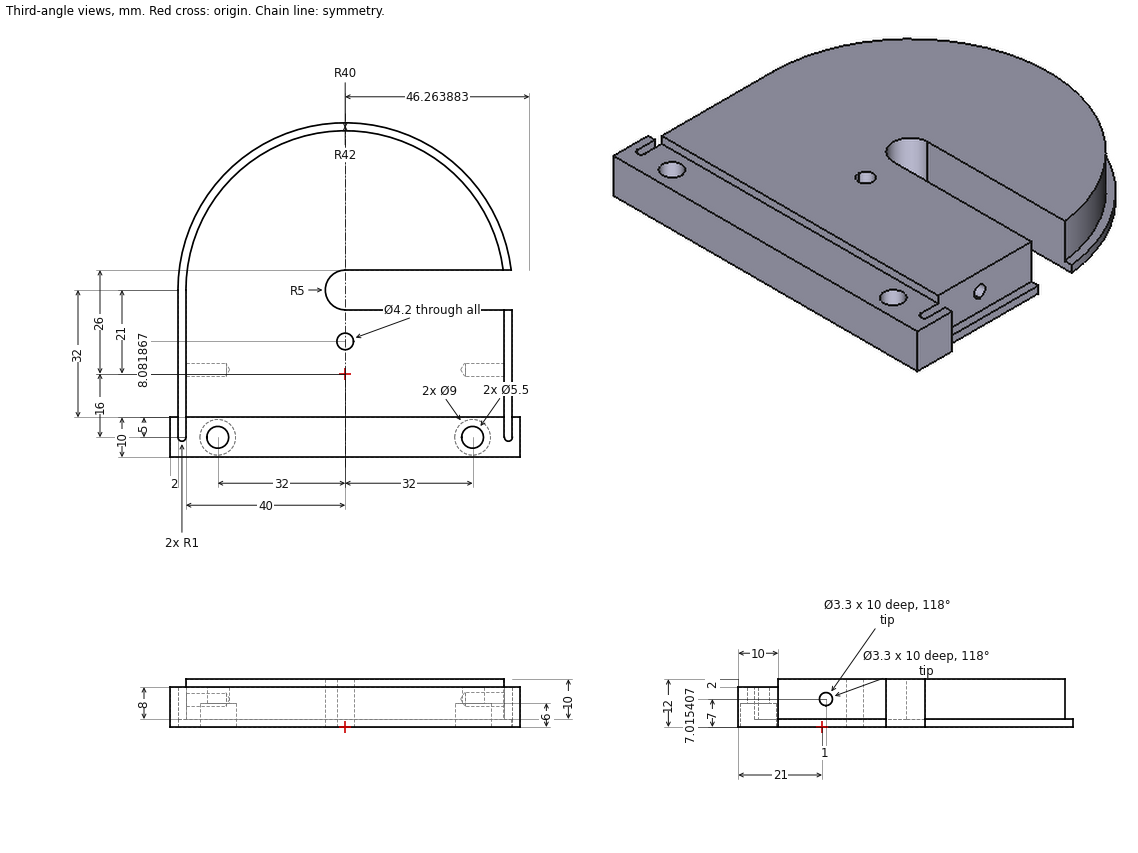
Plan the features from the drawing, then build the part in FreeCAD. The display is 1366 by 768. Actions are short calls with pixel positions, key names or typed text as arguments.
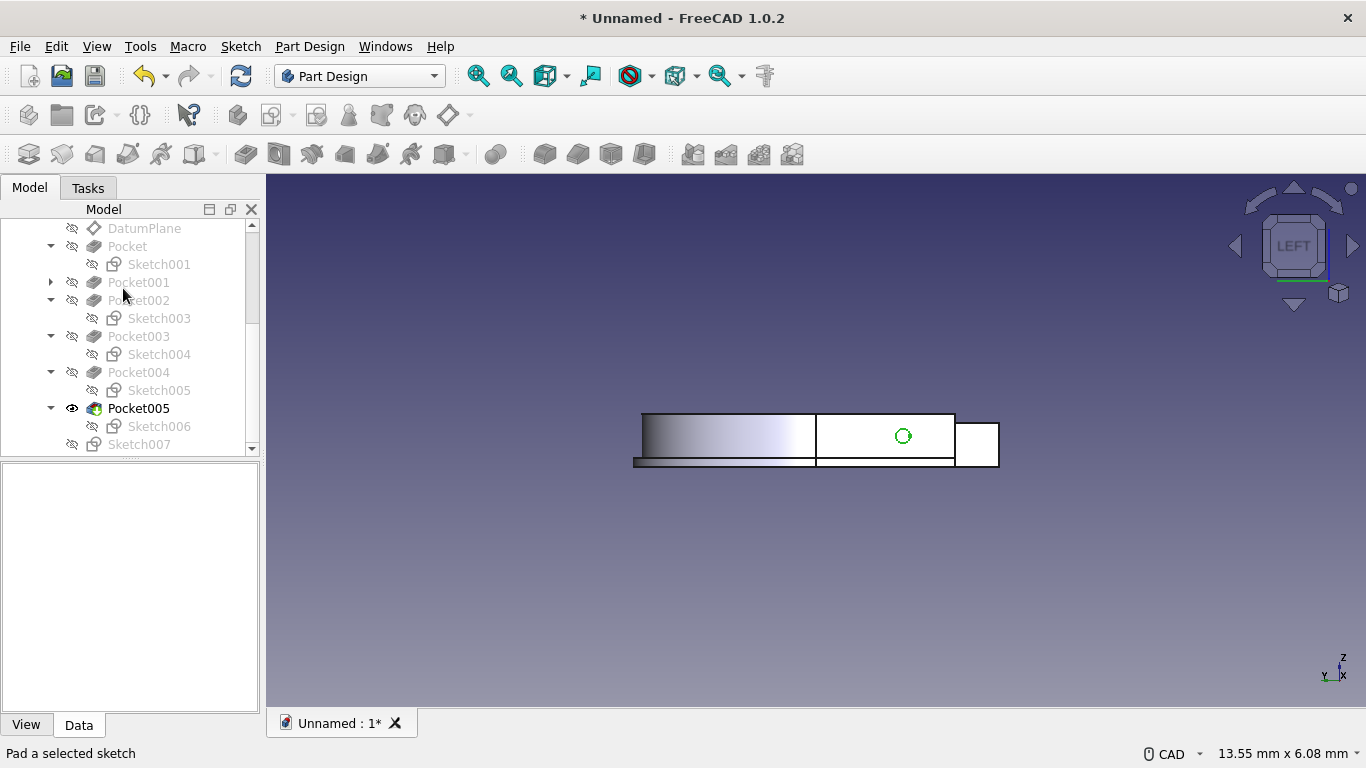
click(279, 154)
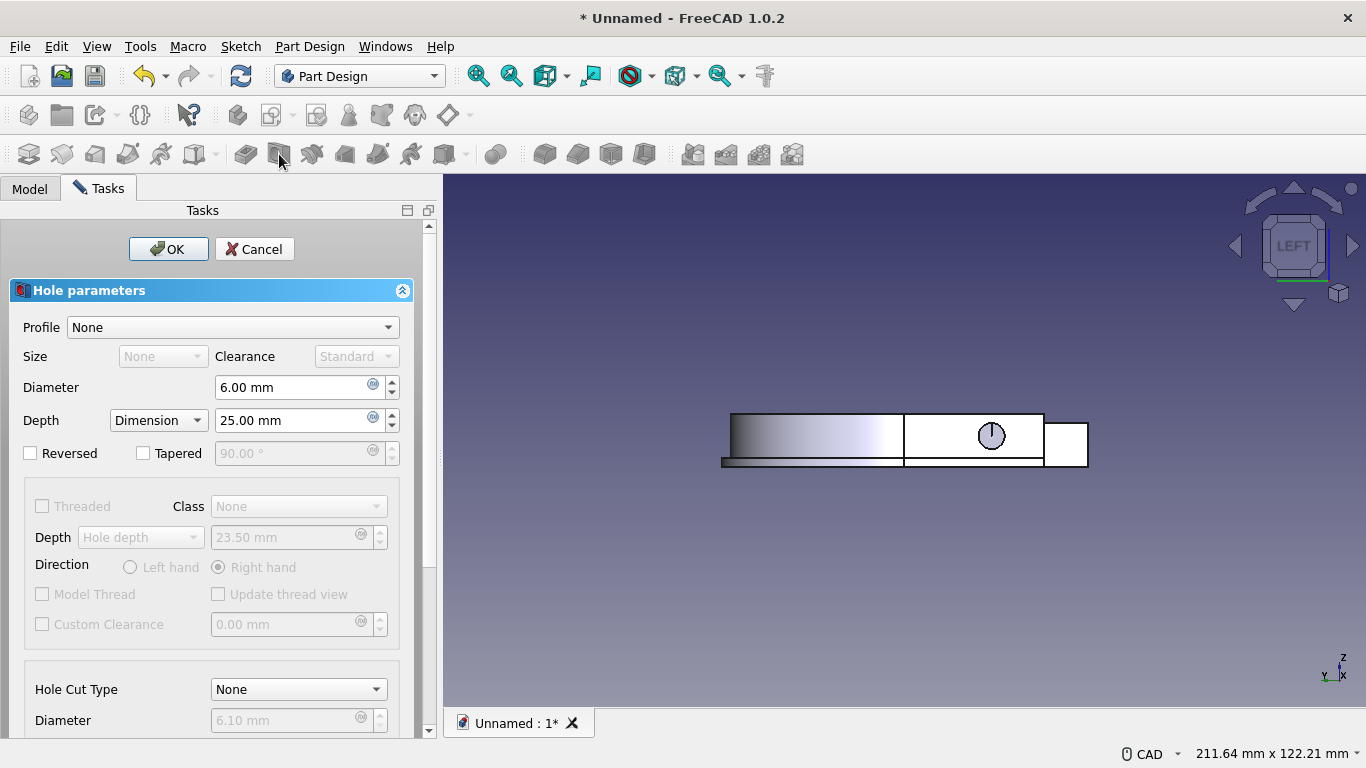
triple_click(300, 388)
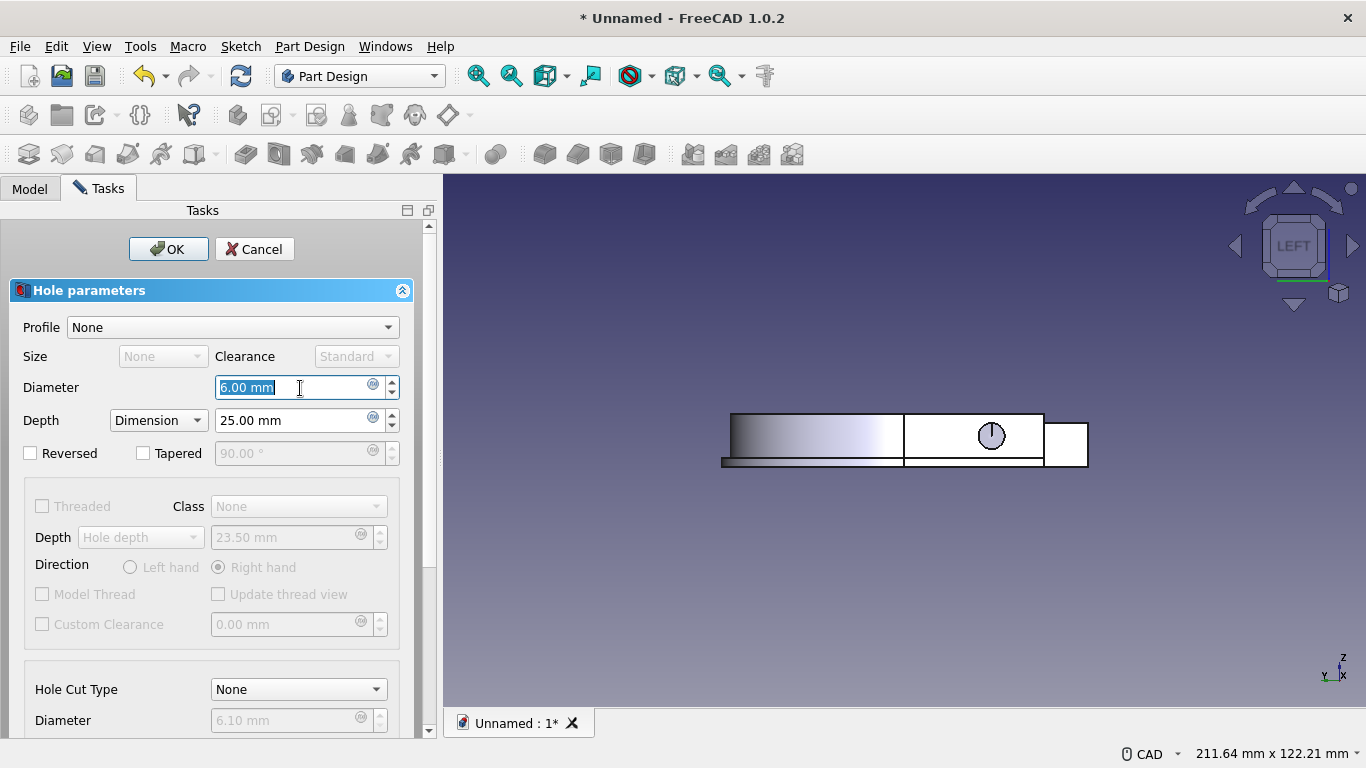
text(3.3)
key(Tab)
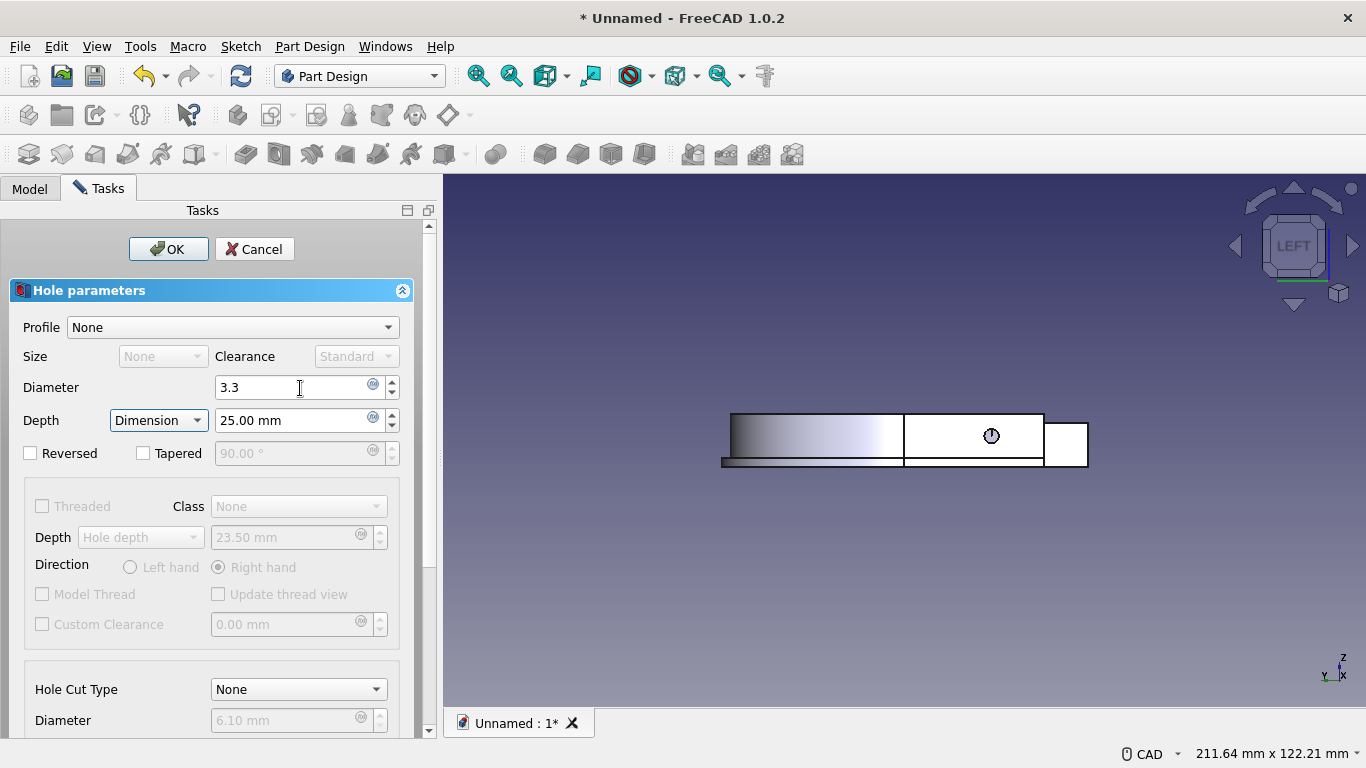
triple_click(300, 420)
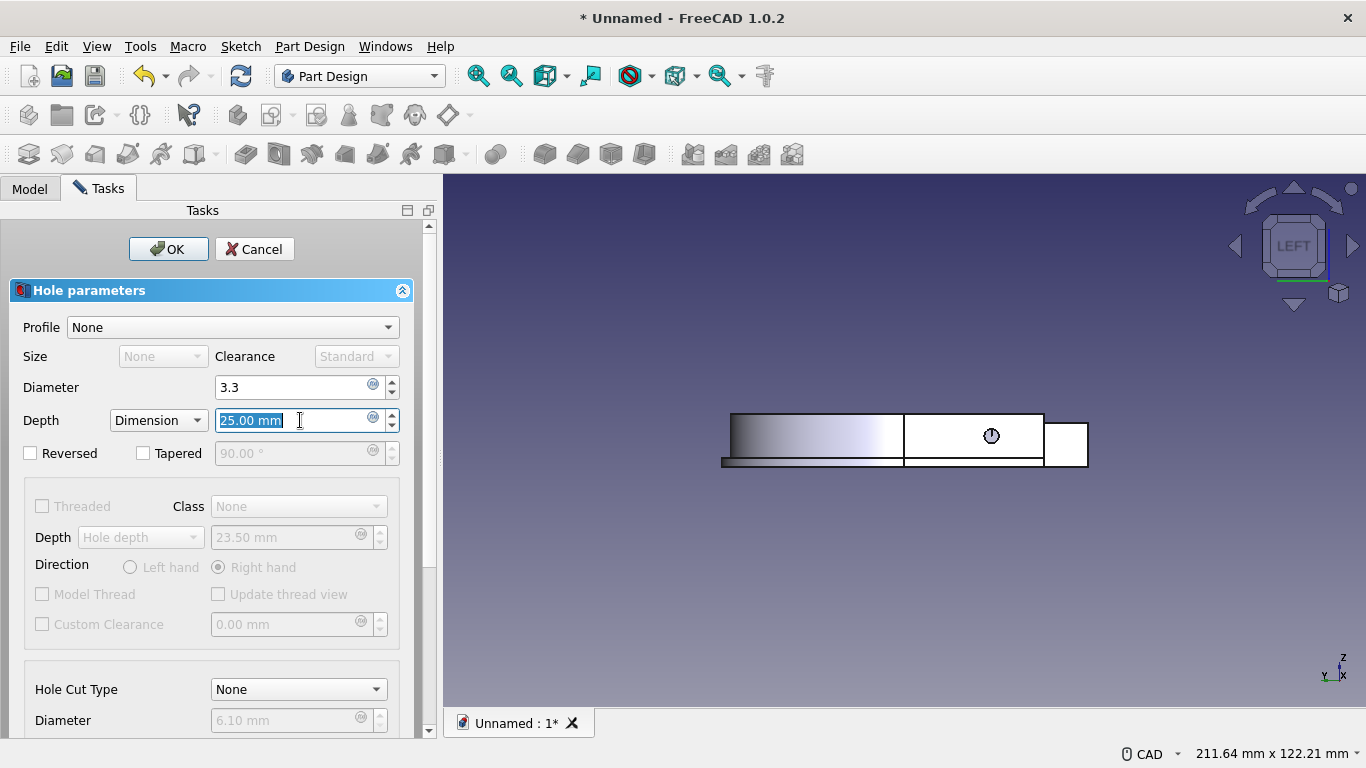
text(10)
key(Tab)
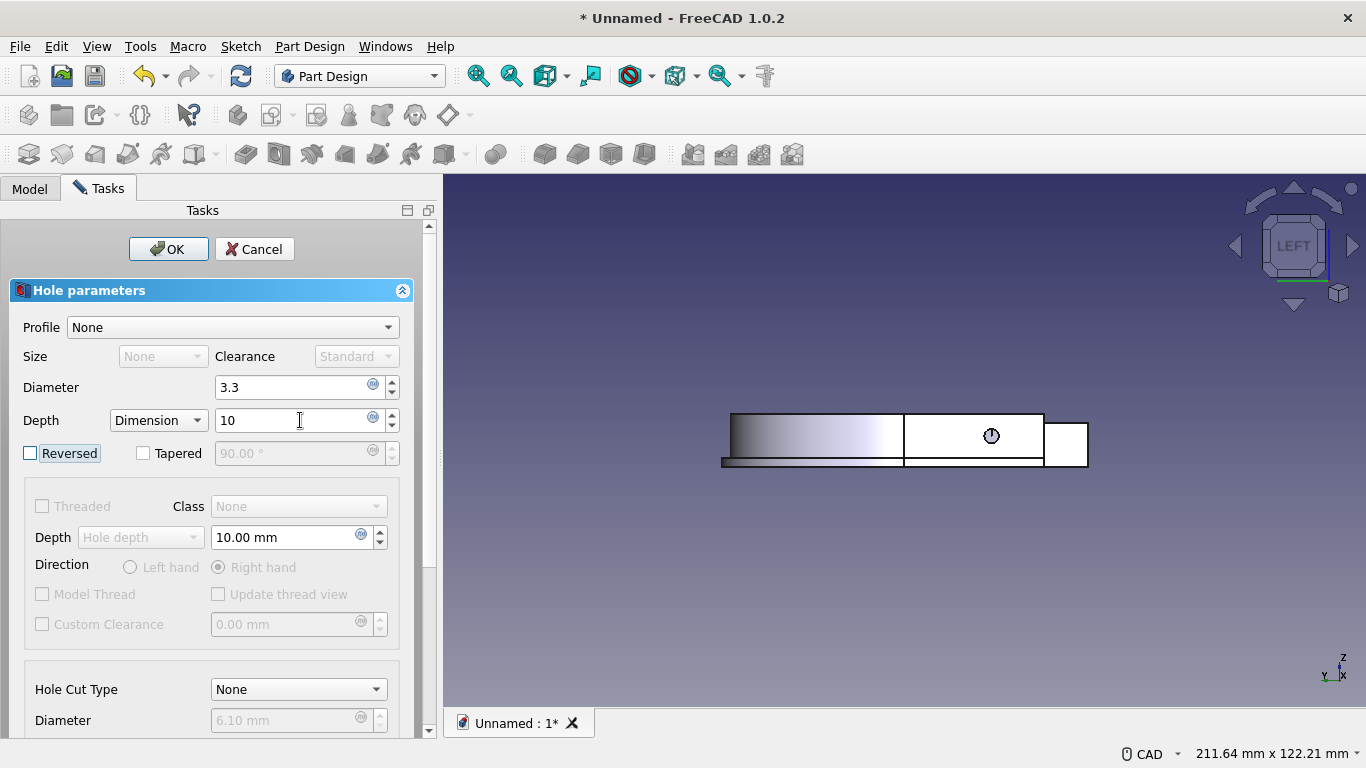
click(169, 249)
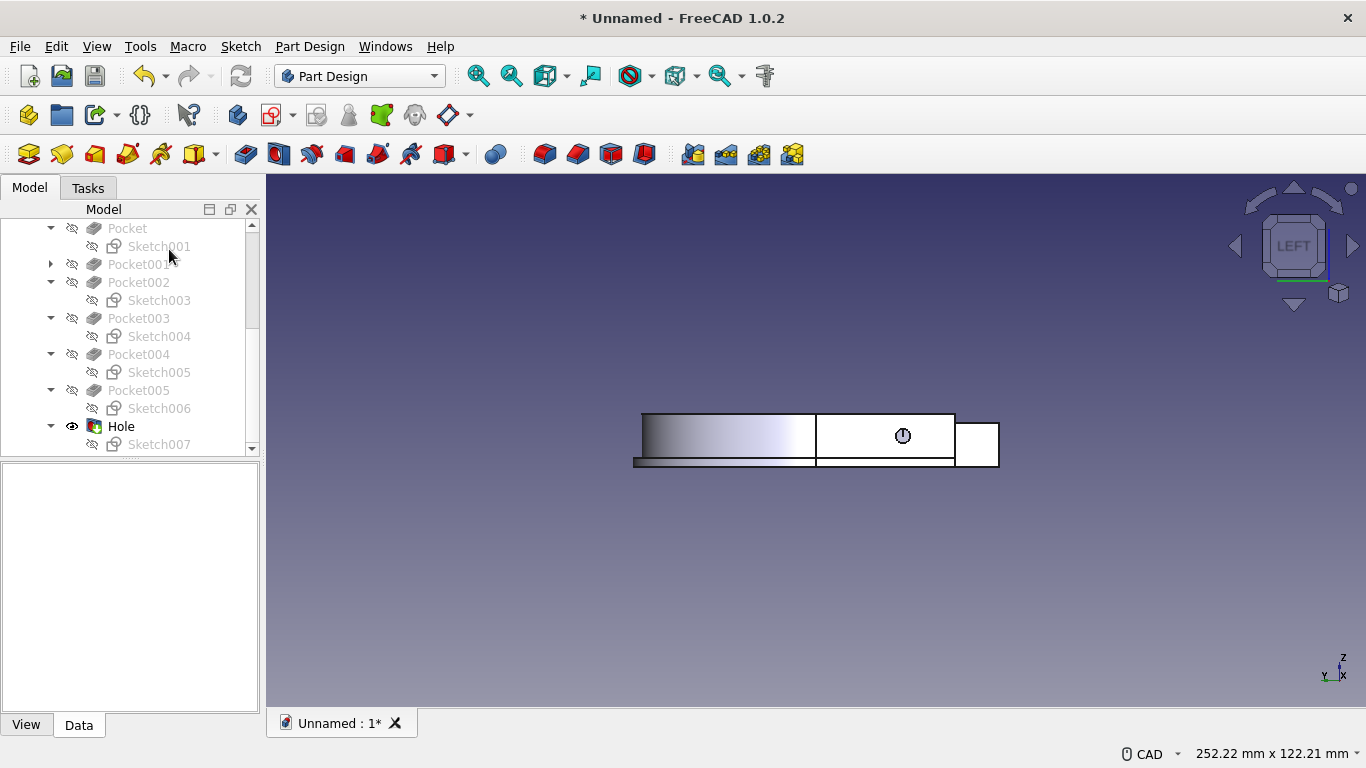
click(479, 76)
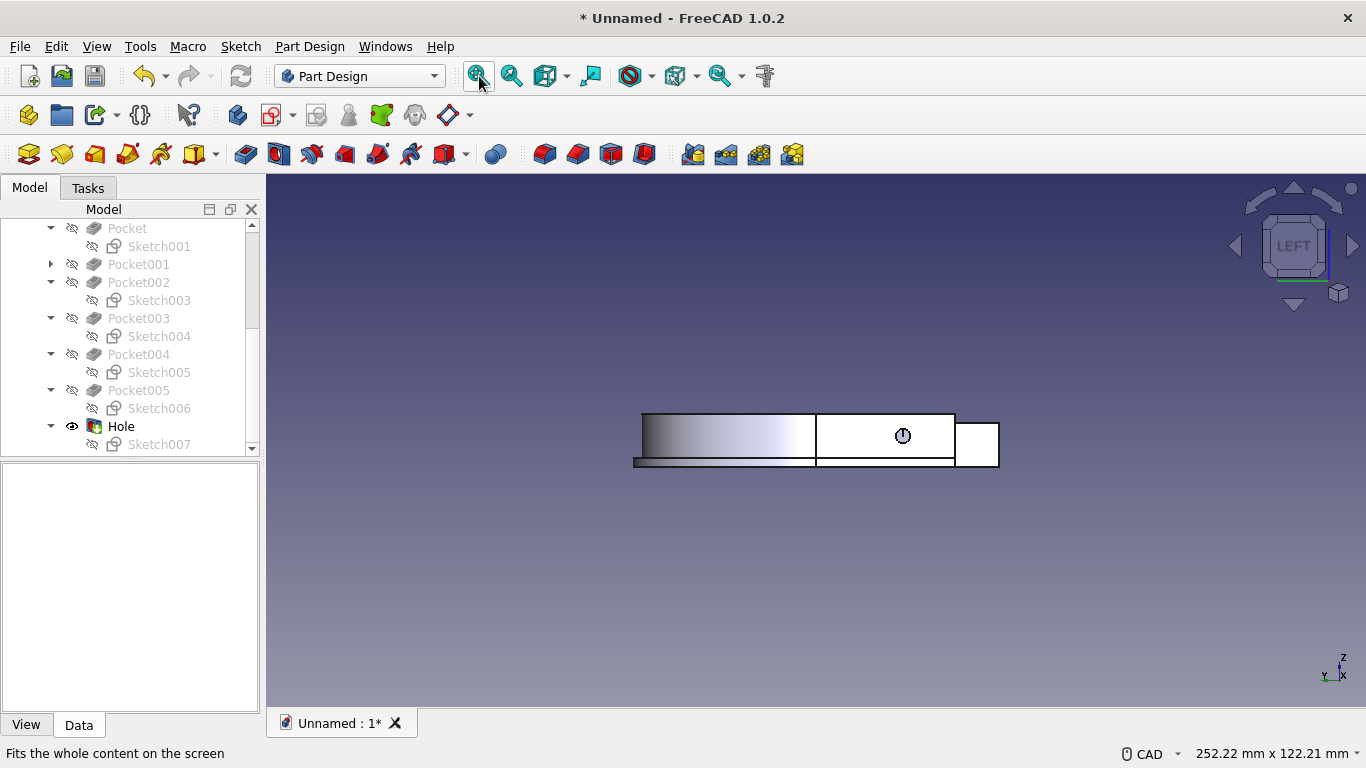
key(0)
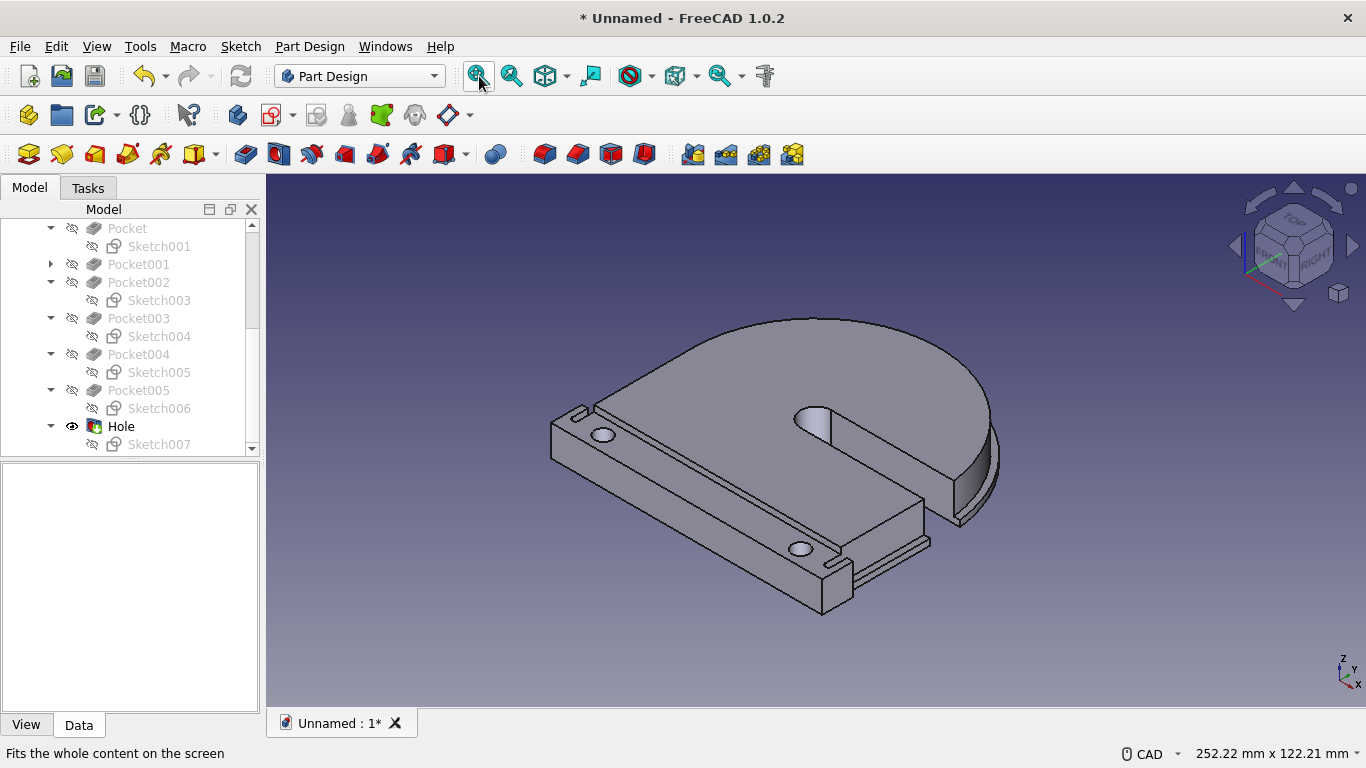
click(861, 553)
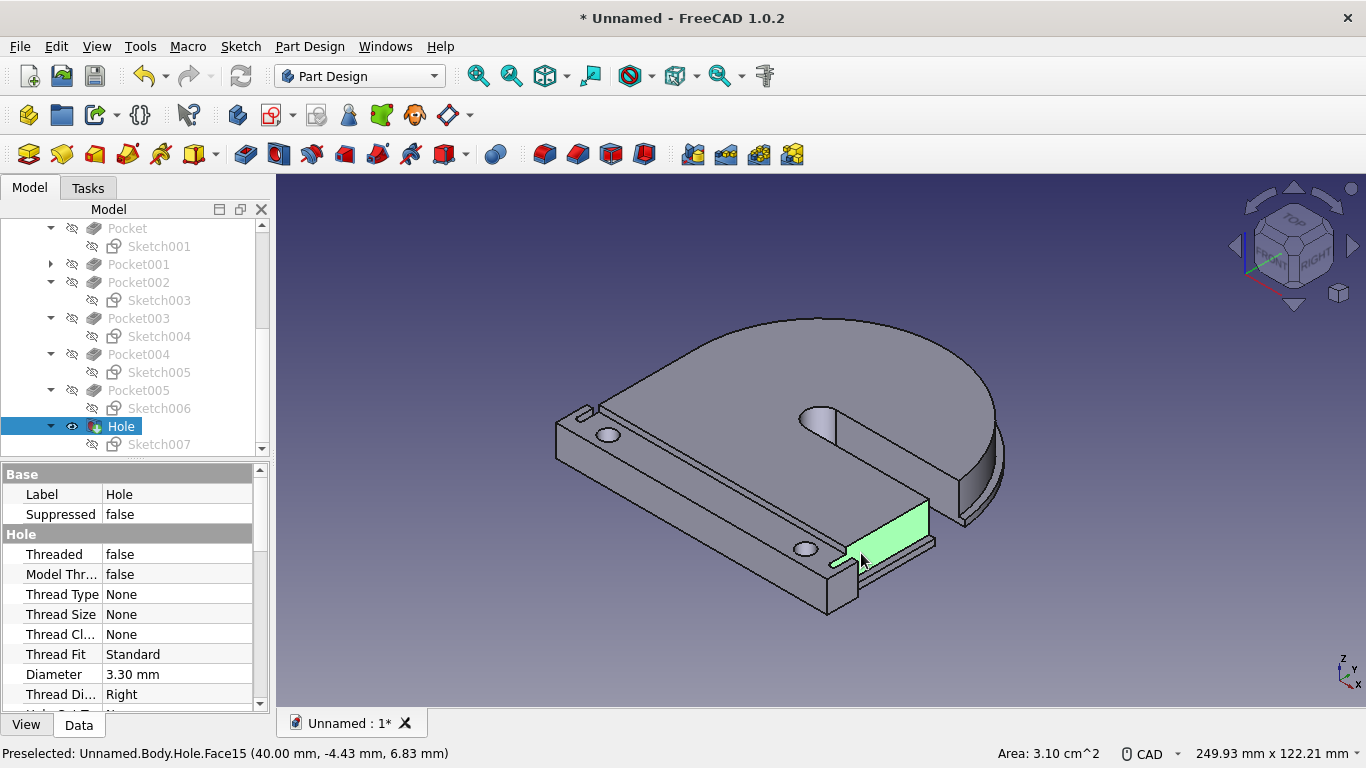
click(270, 116)